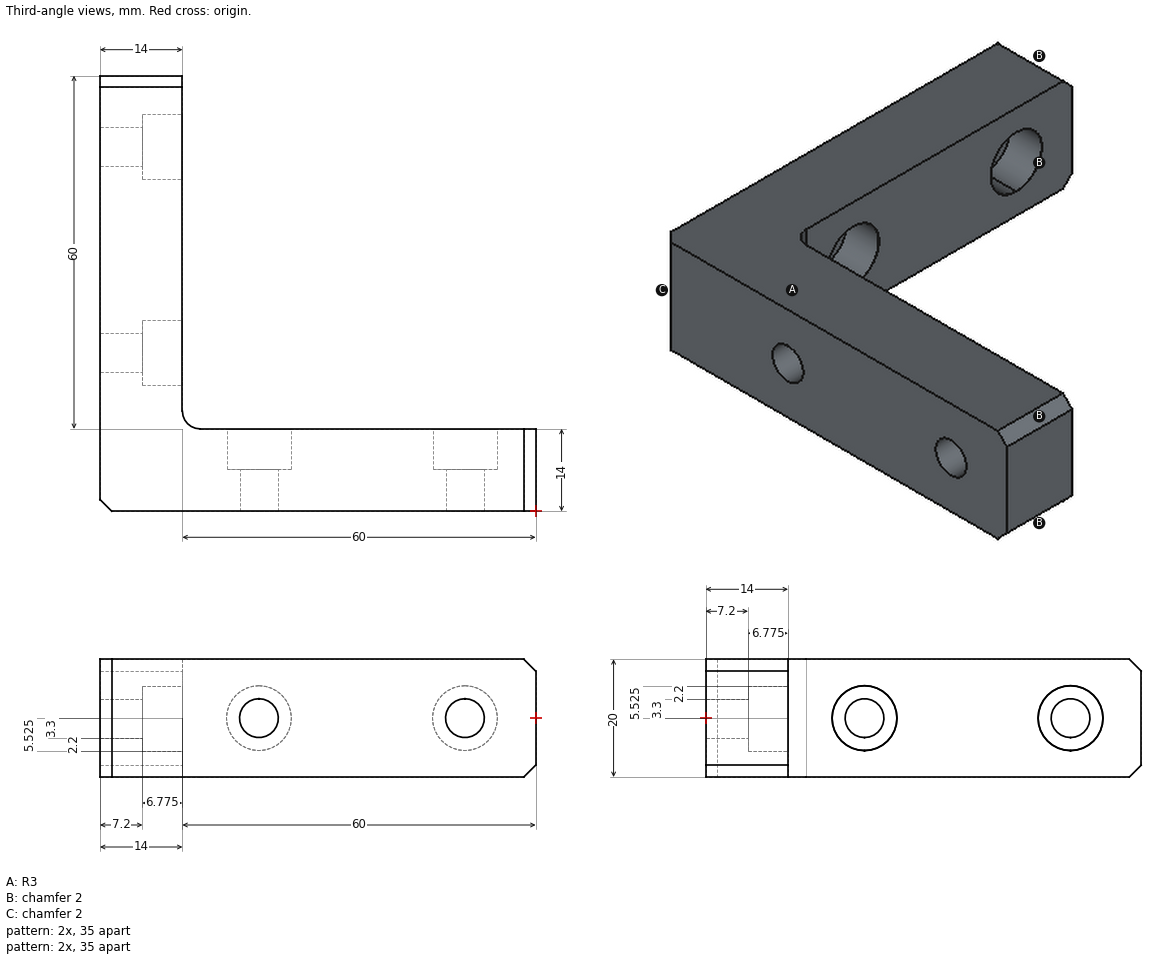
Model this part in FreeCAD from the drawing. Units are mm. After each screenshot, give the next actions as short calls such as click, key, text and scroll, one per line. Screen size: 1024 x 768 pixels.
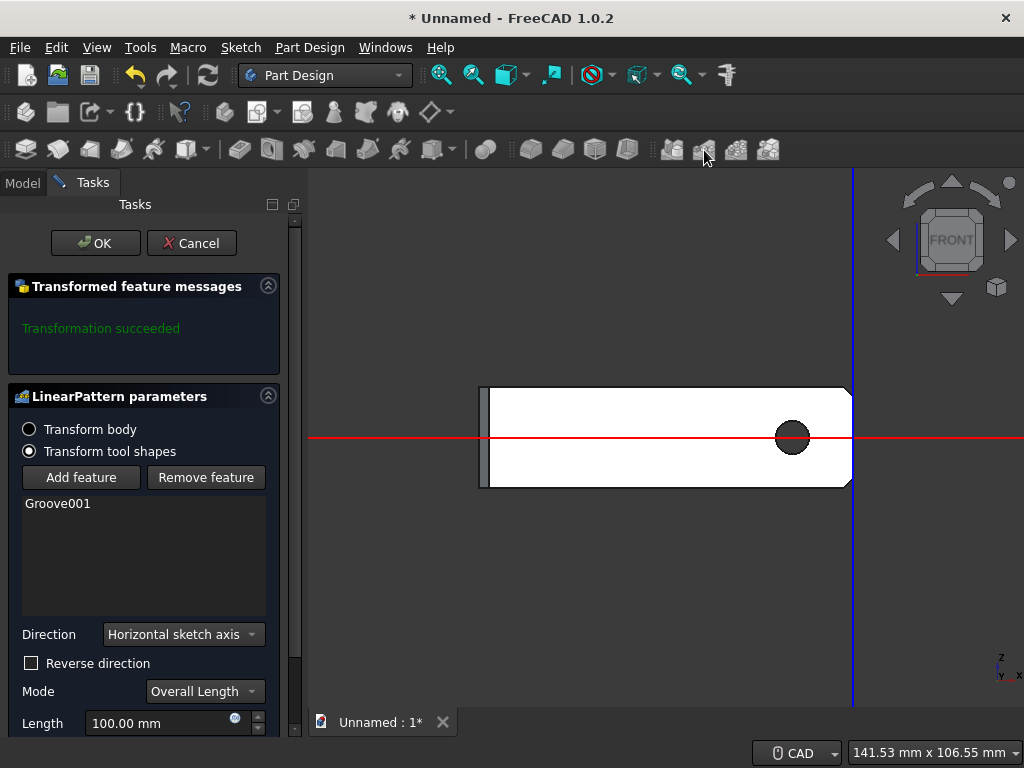
click(184, 634)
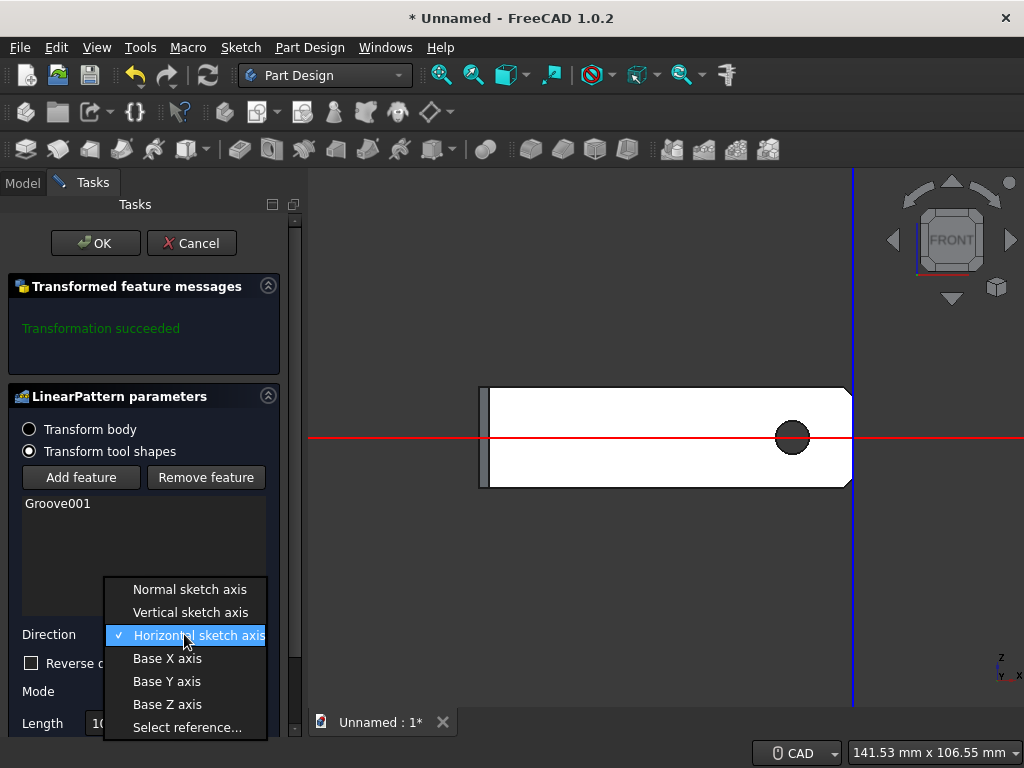
click(184, 658)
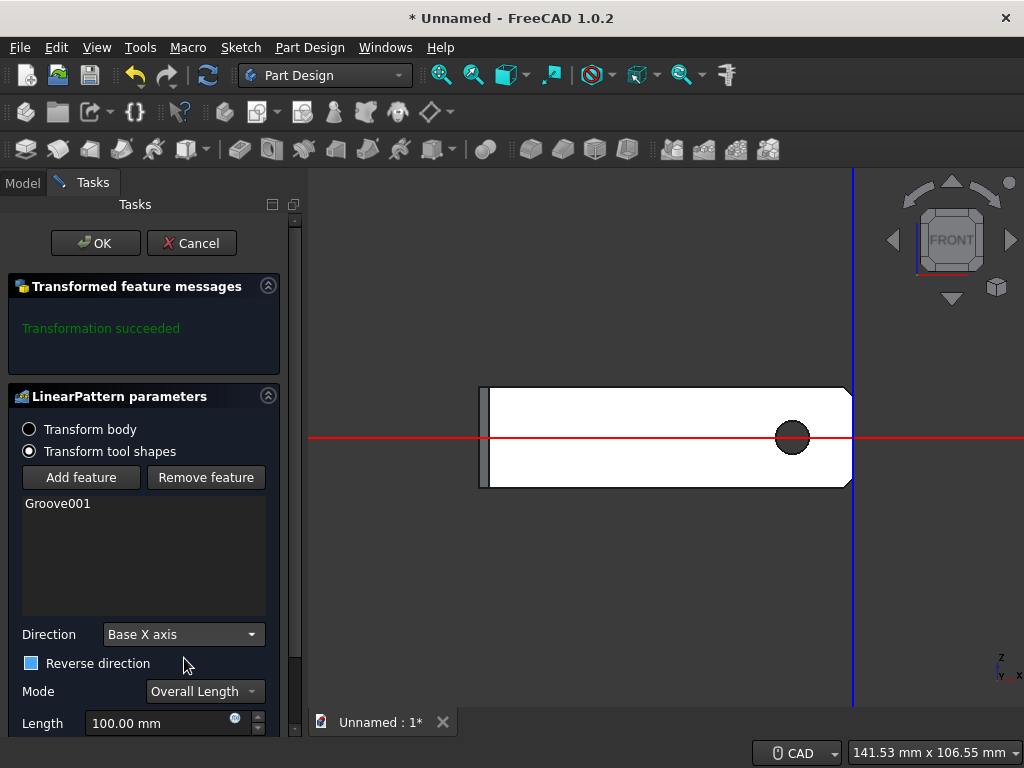
click(206, 692)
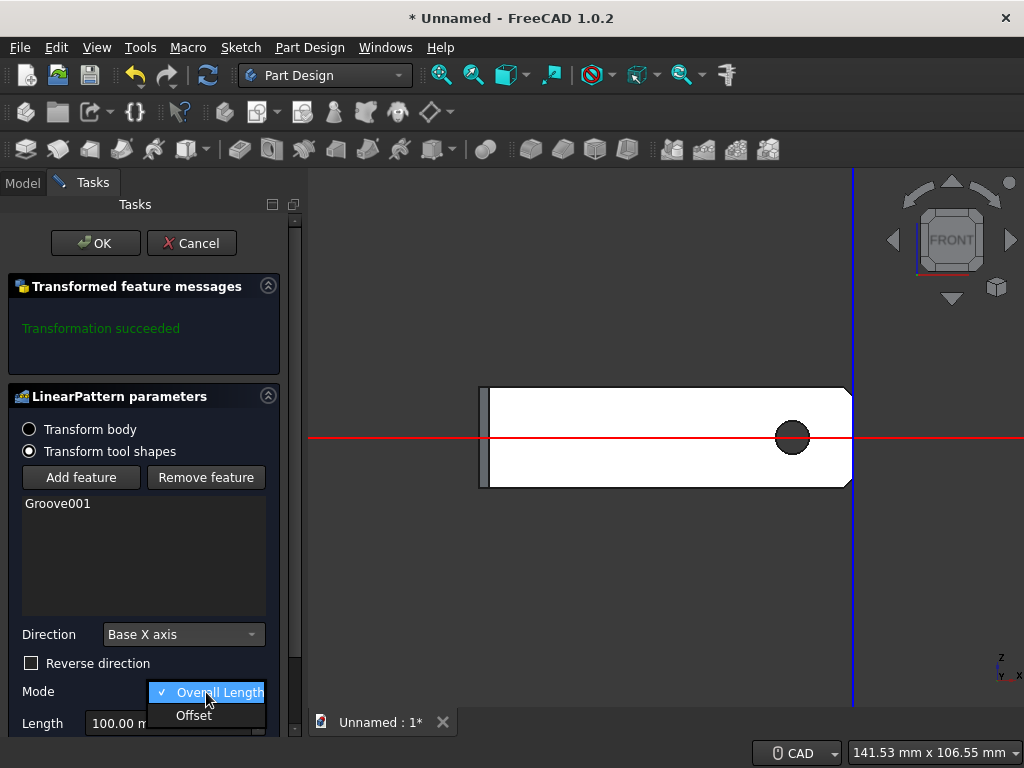
click(206, 716)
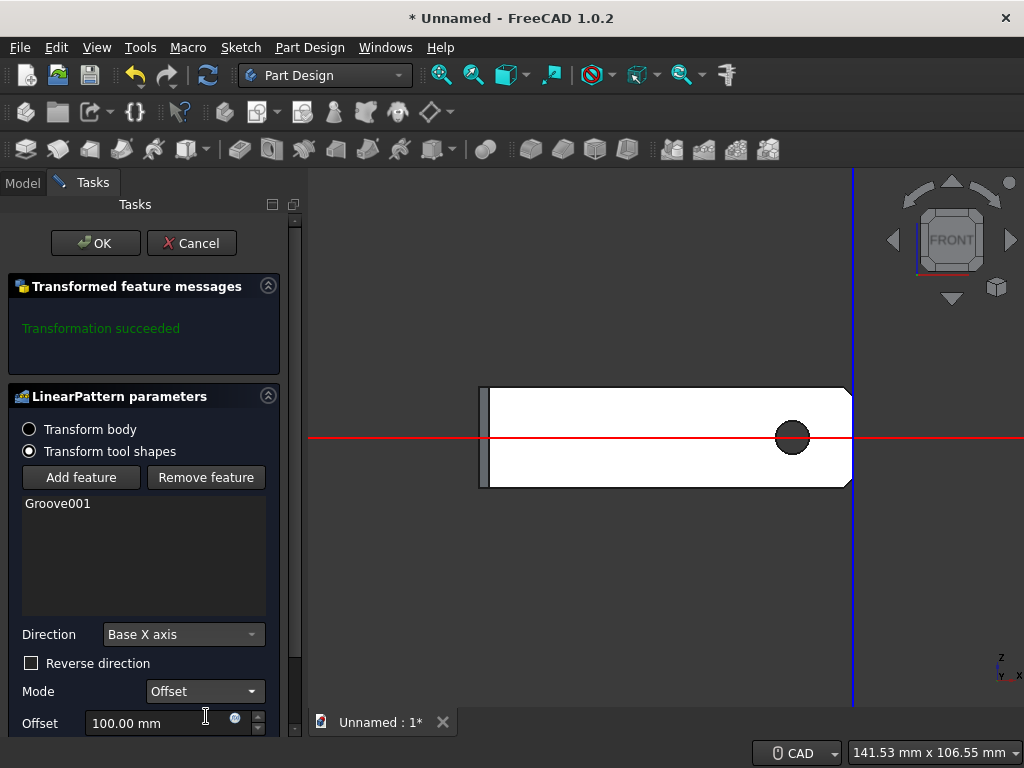
triple_click(168, 723)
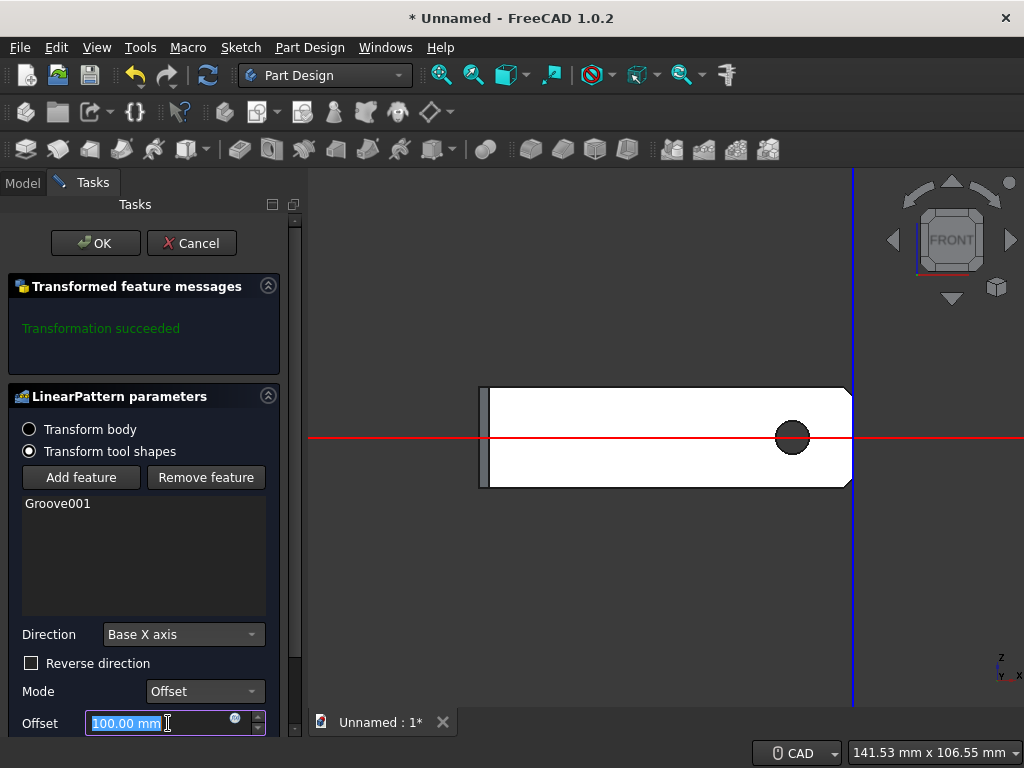
text(35)
key(Tab)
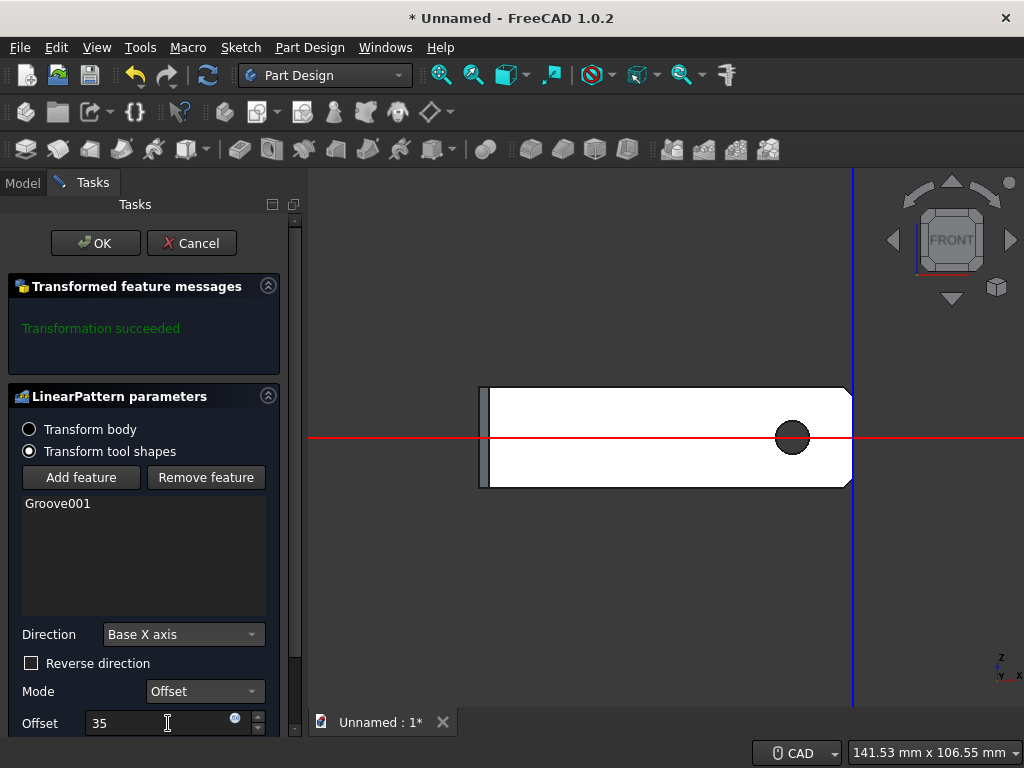
scroll(295, 475, down, 2)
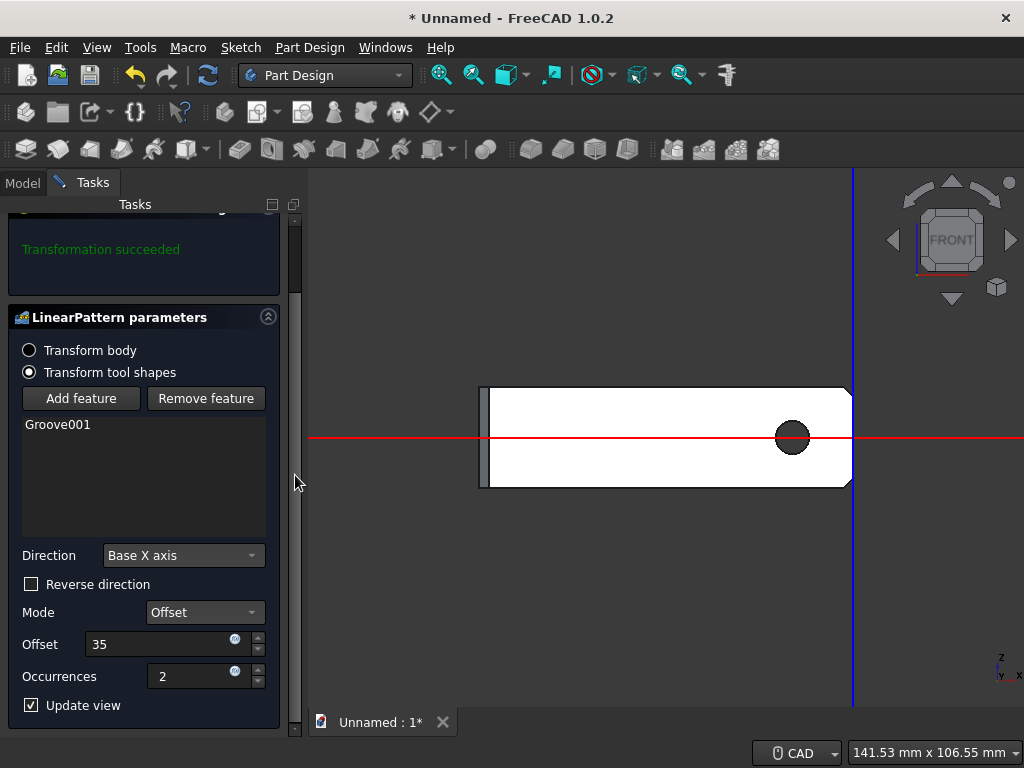
triple_click(198, 676)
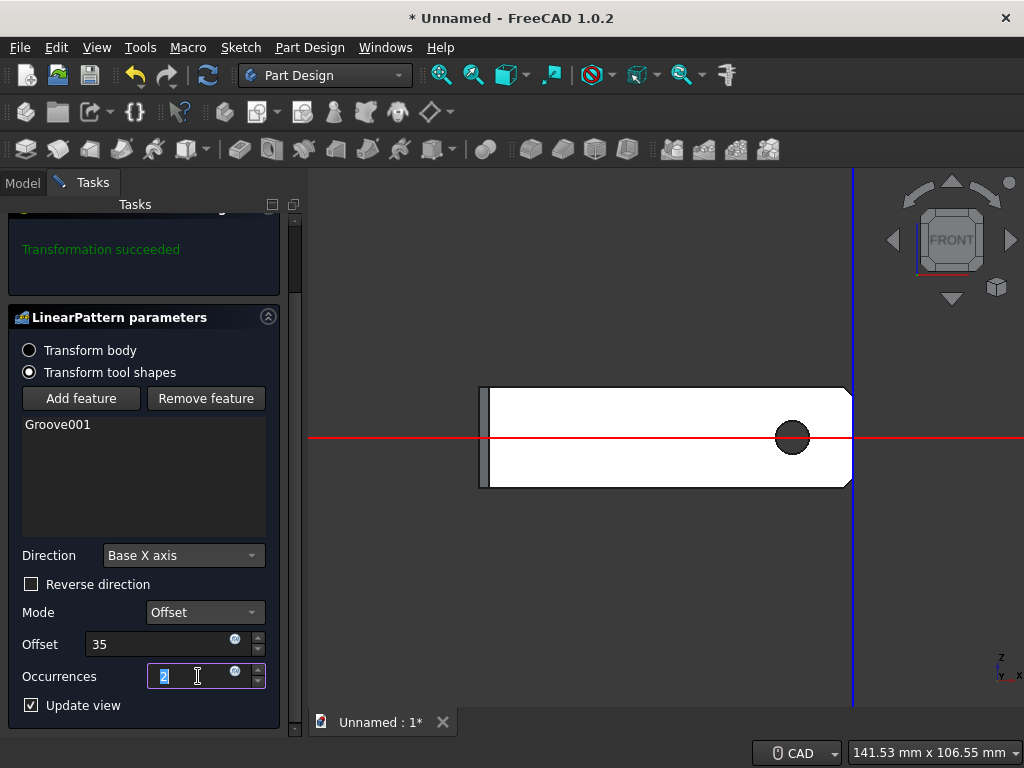
text(2)
key(Tab)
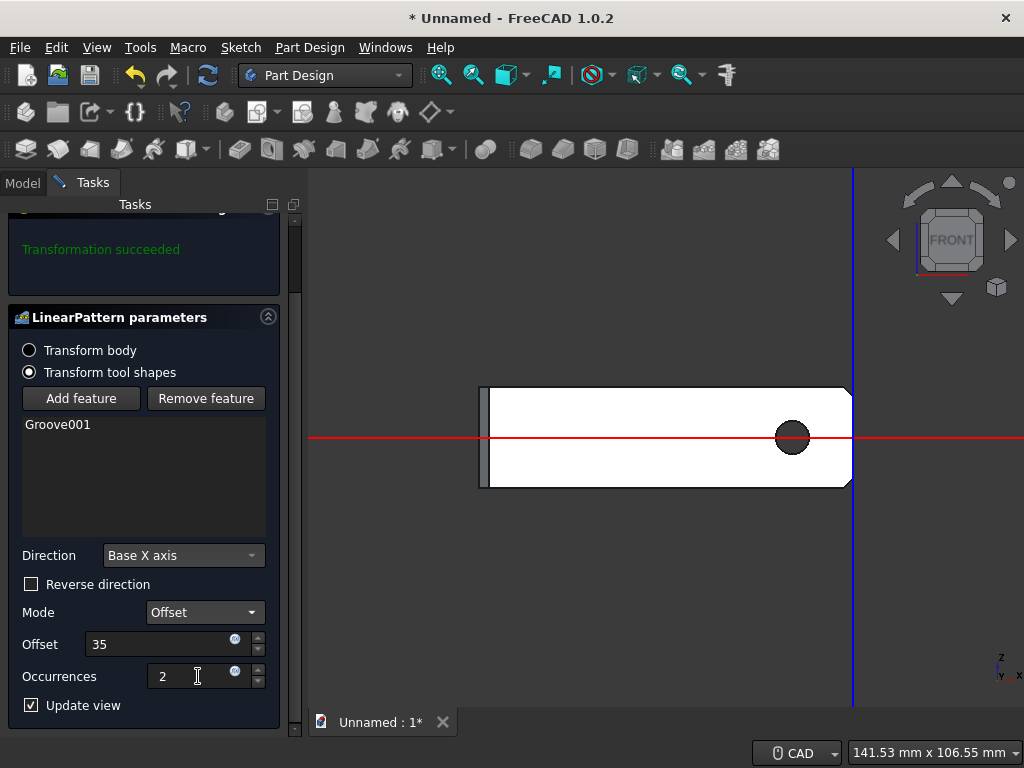
click(30, 584)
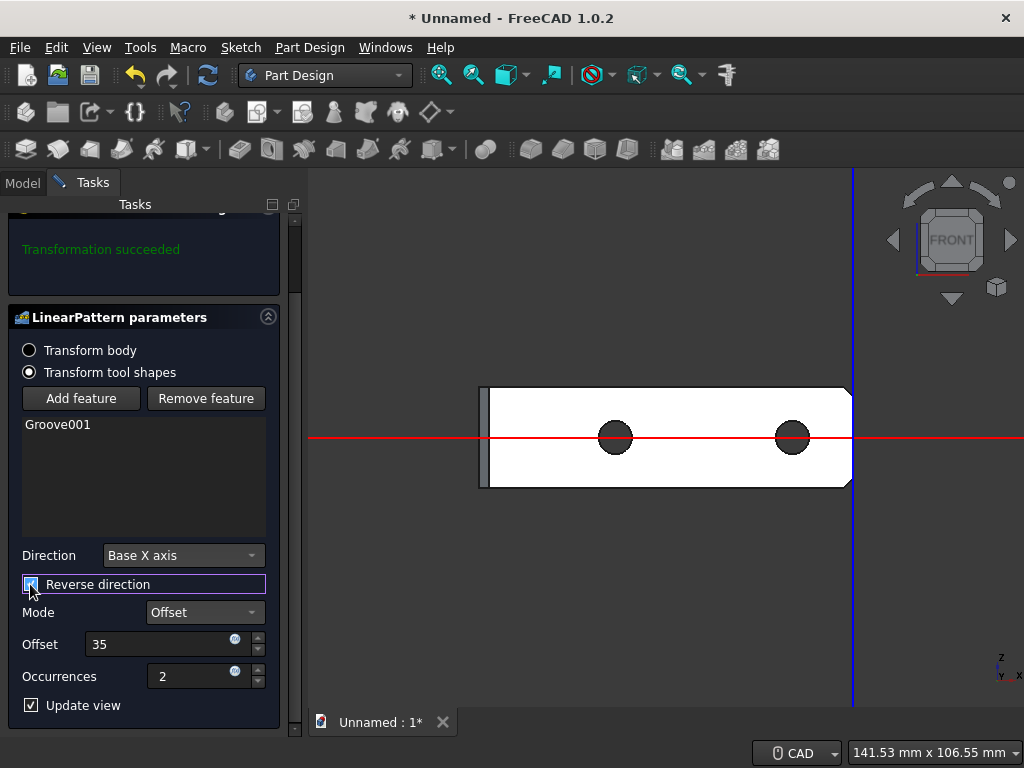
scroll(295, 475, up, 3)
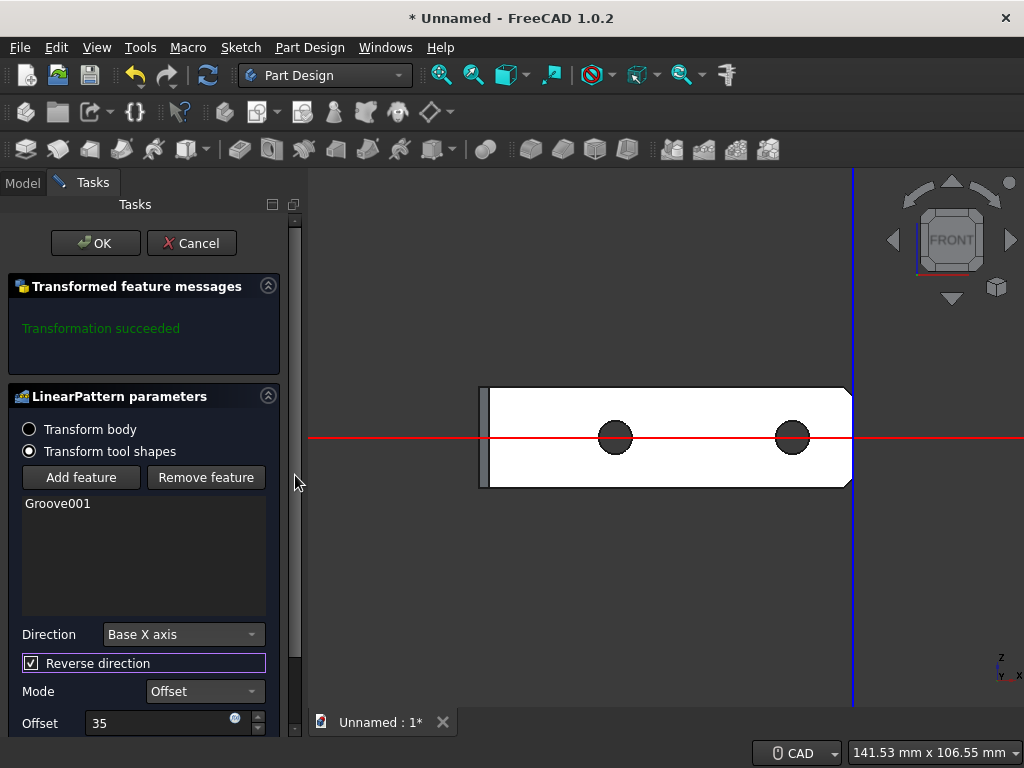
click(96, 243)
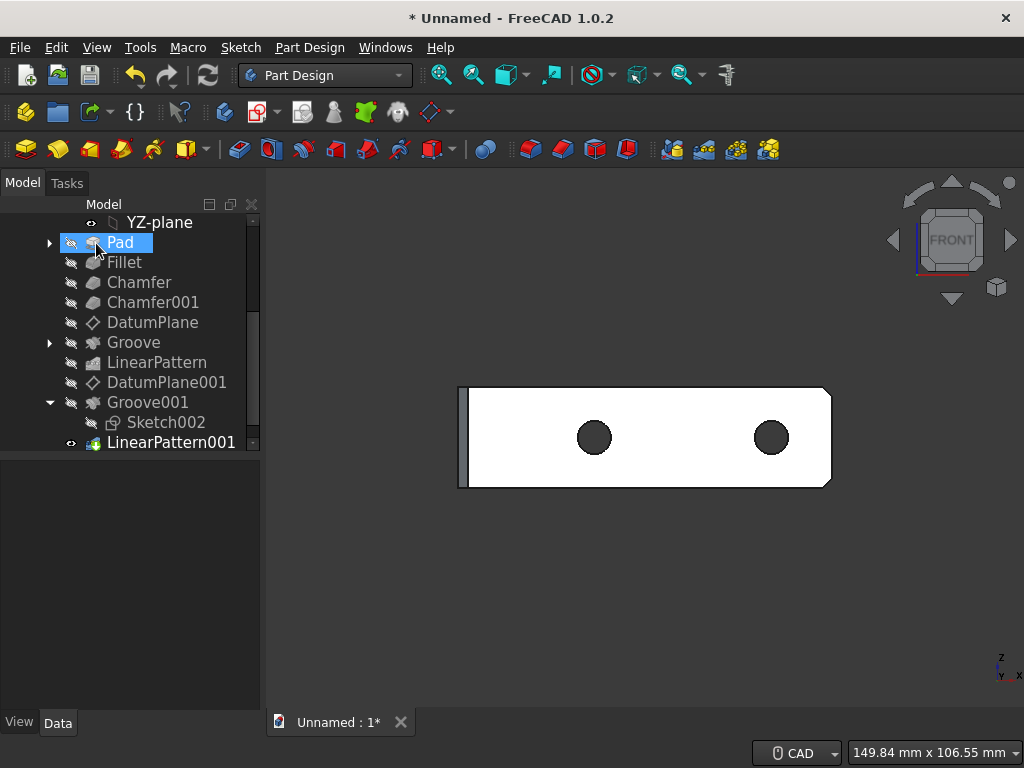
key(0)